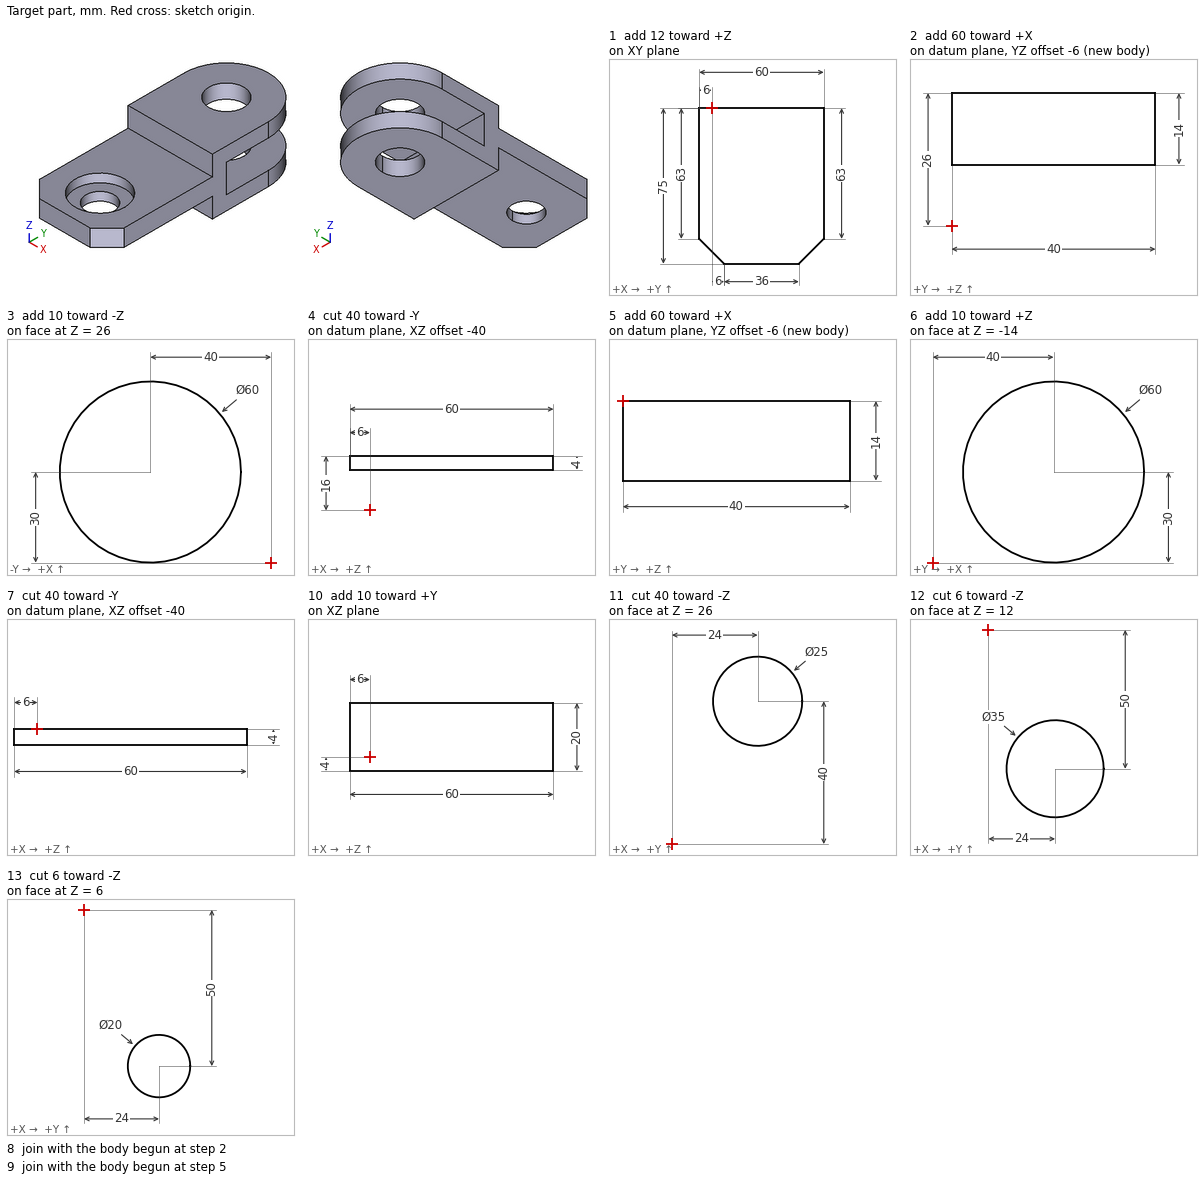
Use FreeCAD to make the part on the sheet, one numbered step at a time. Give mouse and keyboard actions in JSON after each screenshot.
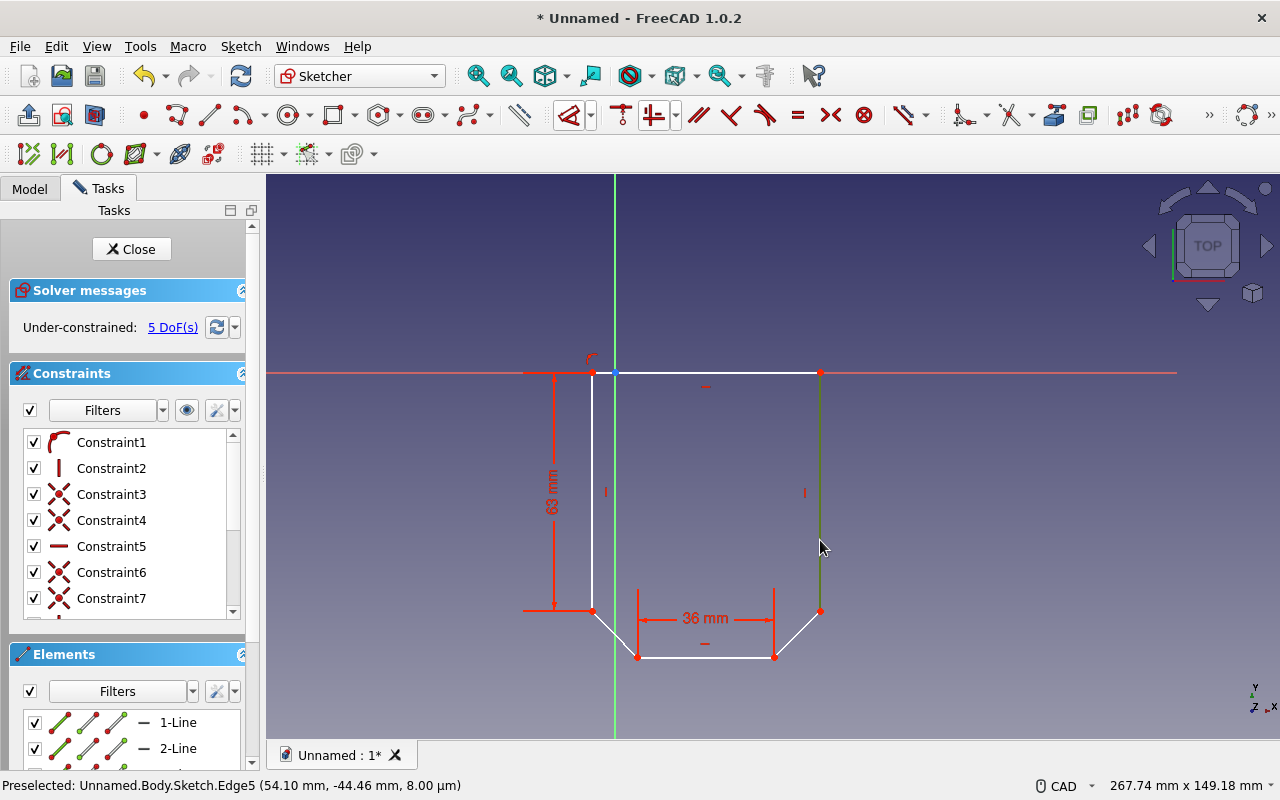
{"action": "left_click", "coordinate": [590, 116]}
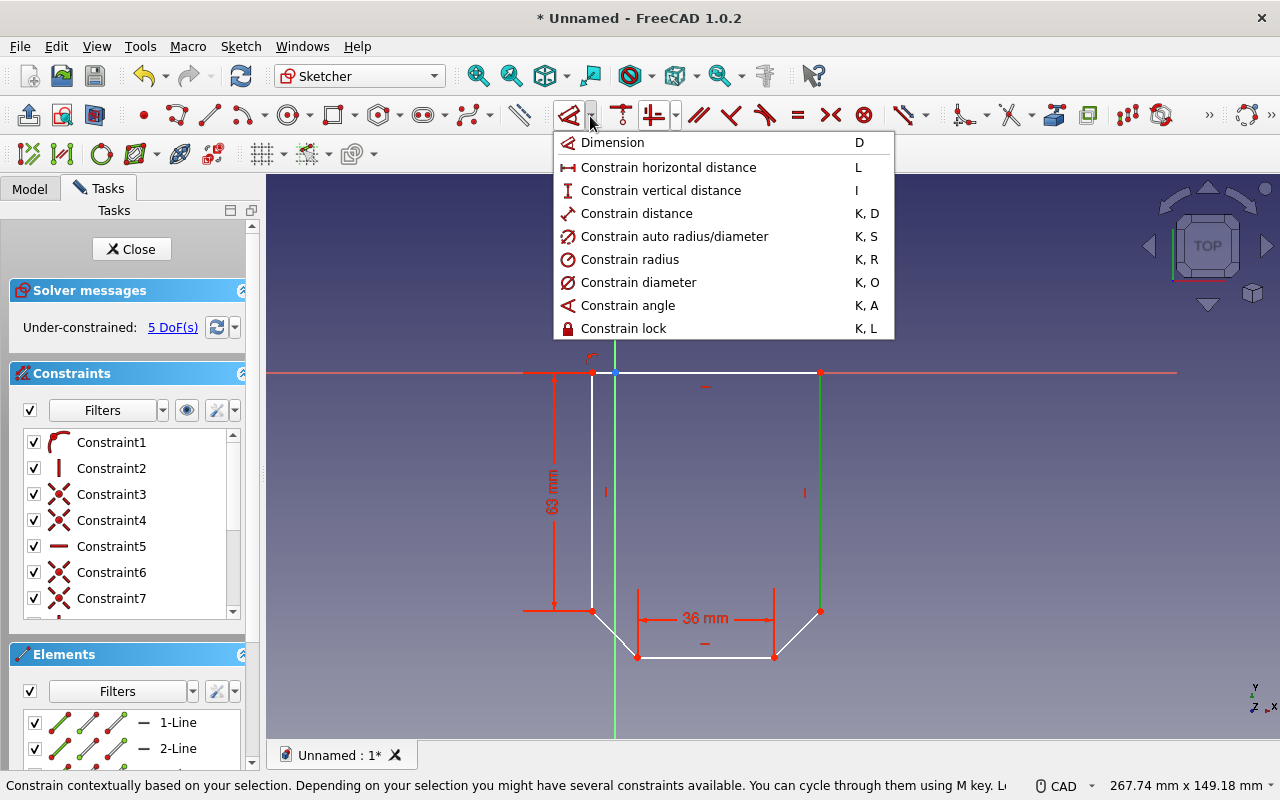
{"action": "left_click", "coordinate": [724, 190]}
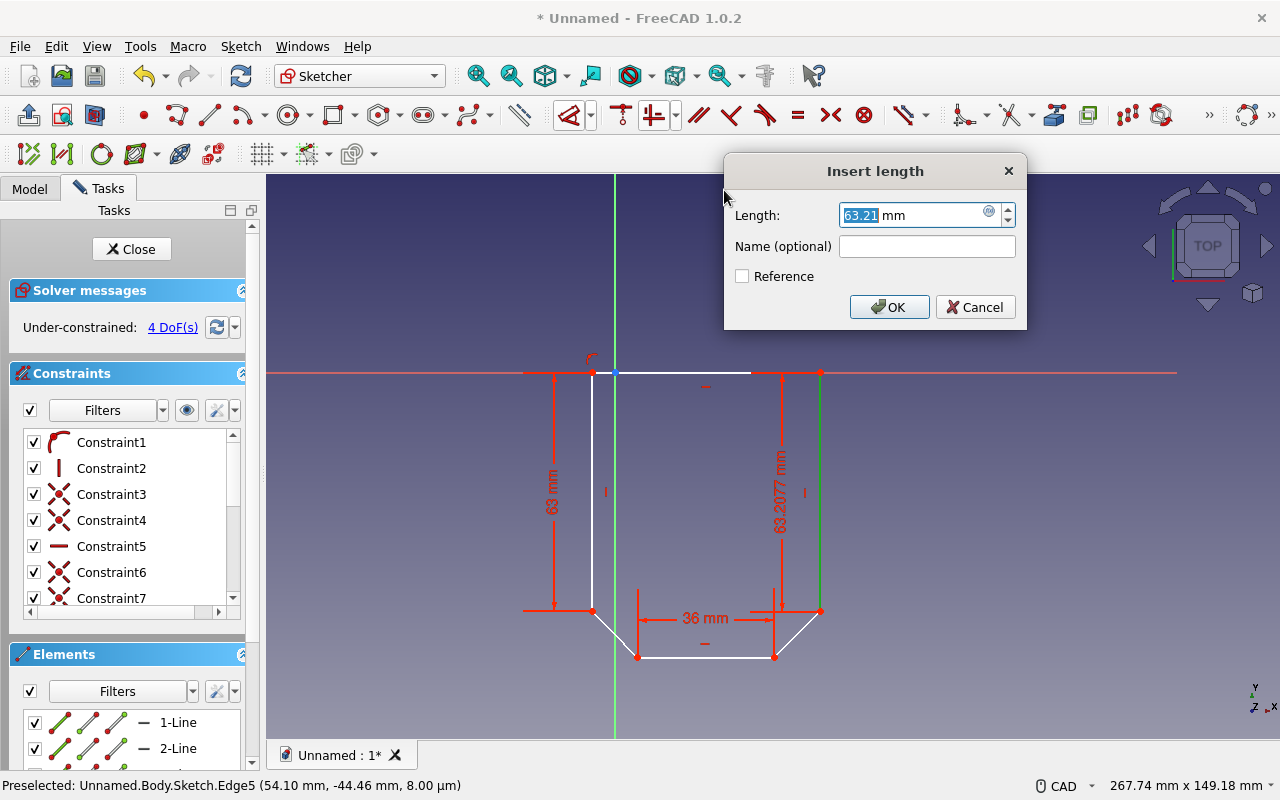
{"action": "type", "text": "63"}
{"action": "key", "text": "Return"}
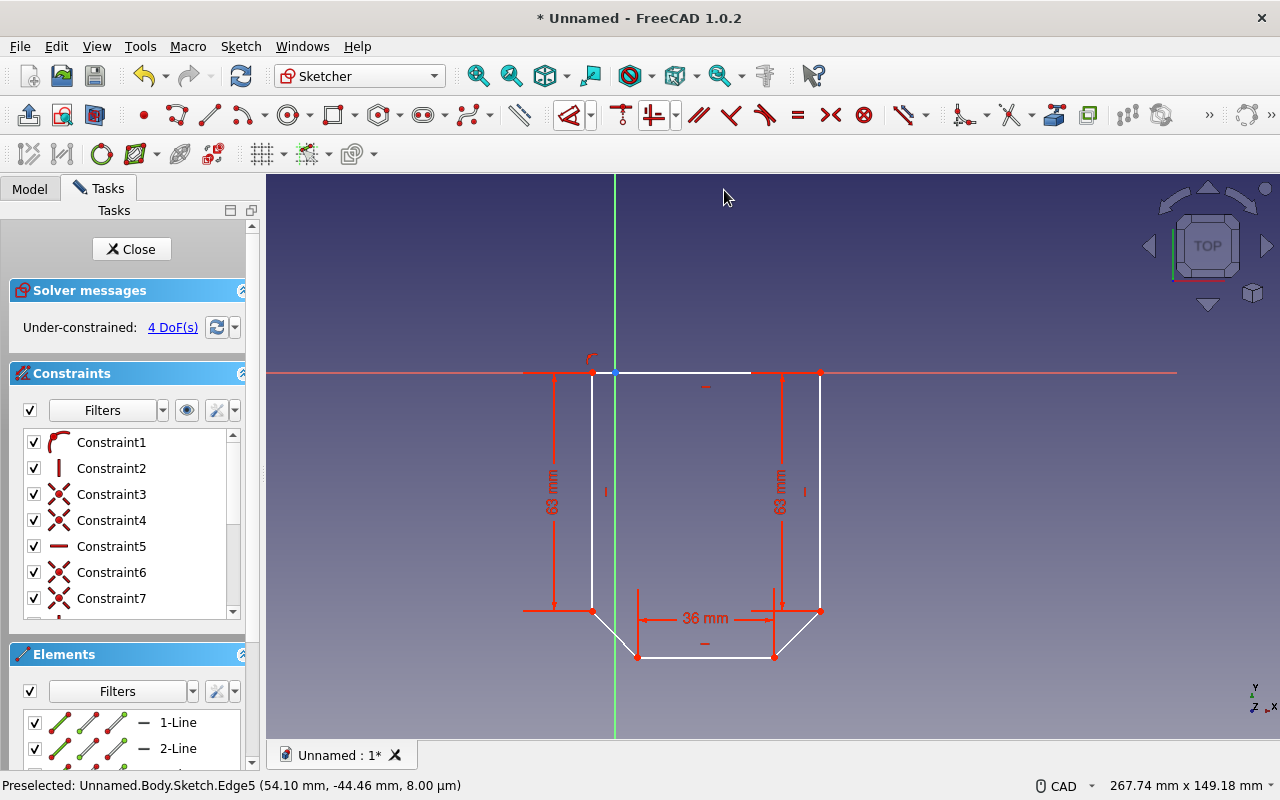
{"action": "left_click", "coordinate": [752, 373]}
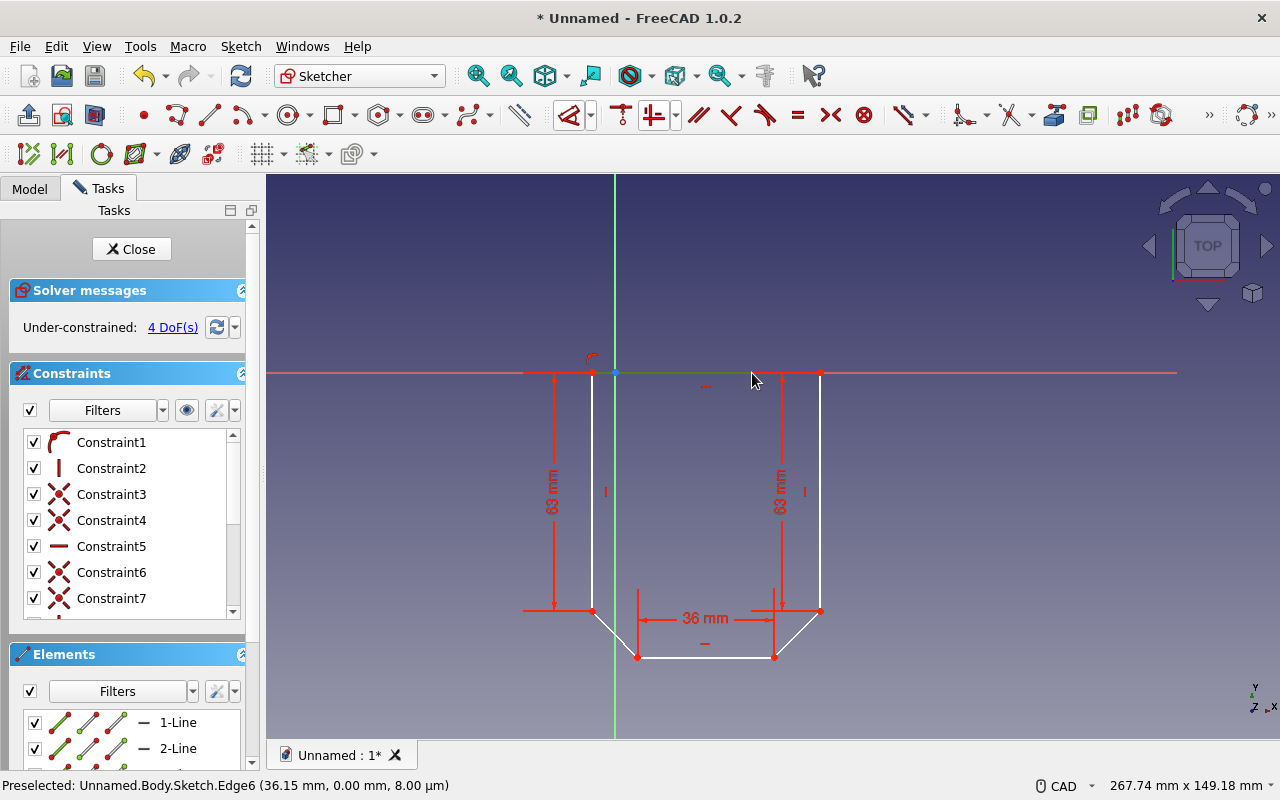
{"action": "left_click", "coordinate": [590, 116]}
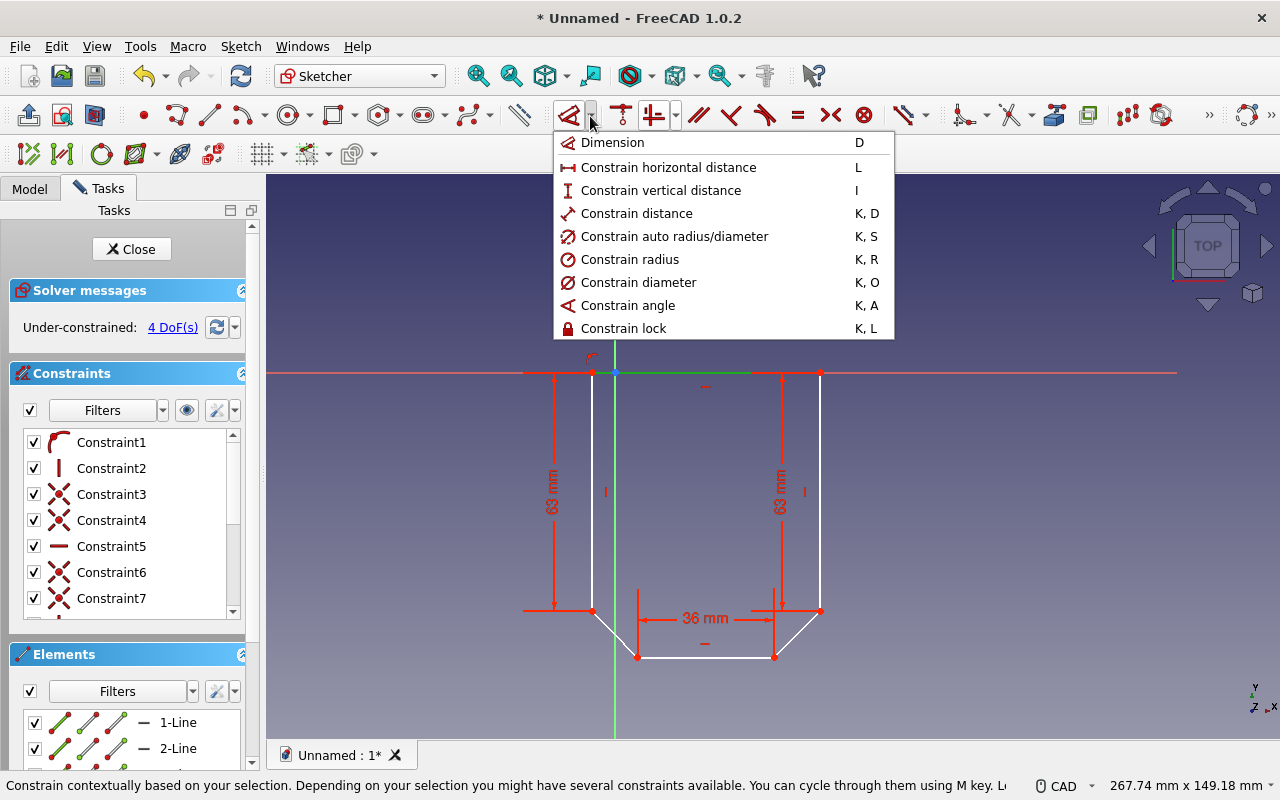
{"action": "left_click", "coordinate": [724, 168]}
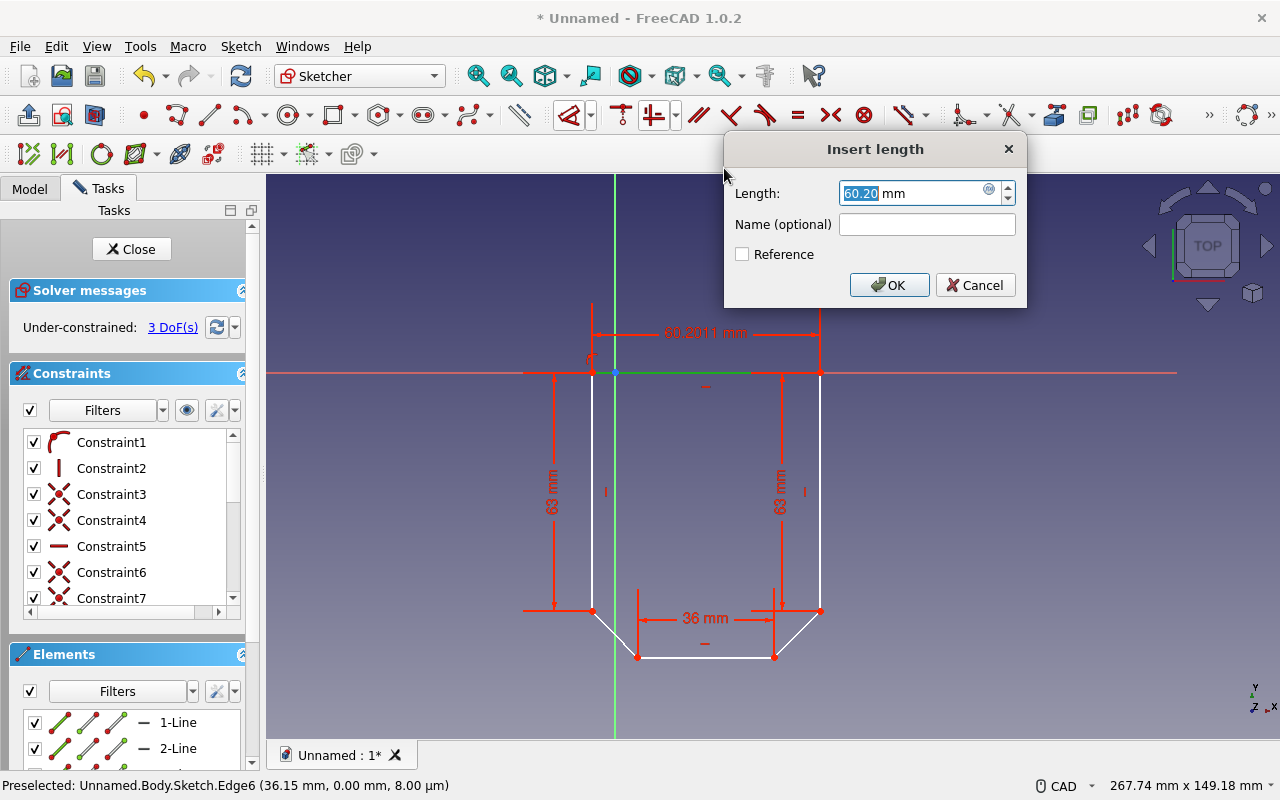
{"action": "type", "text": "60"}
{"action": "key", "text": "Return"}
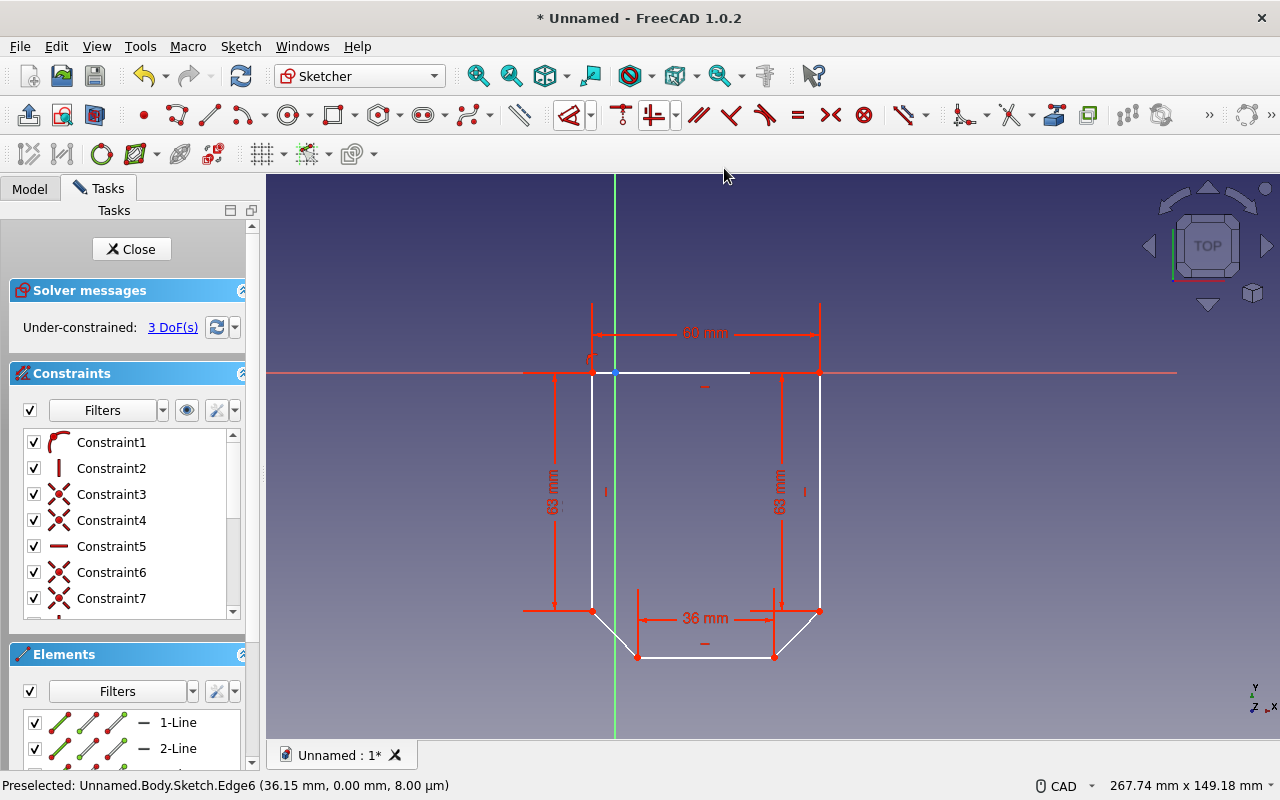
{"action": "scroll", "coordinate": [592, 373], "scroll_direction": "up", "scroll_amount": 3}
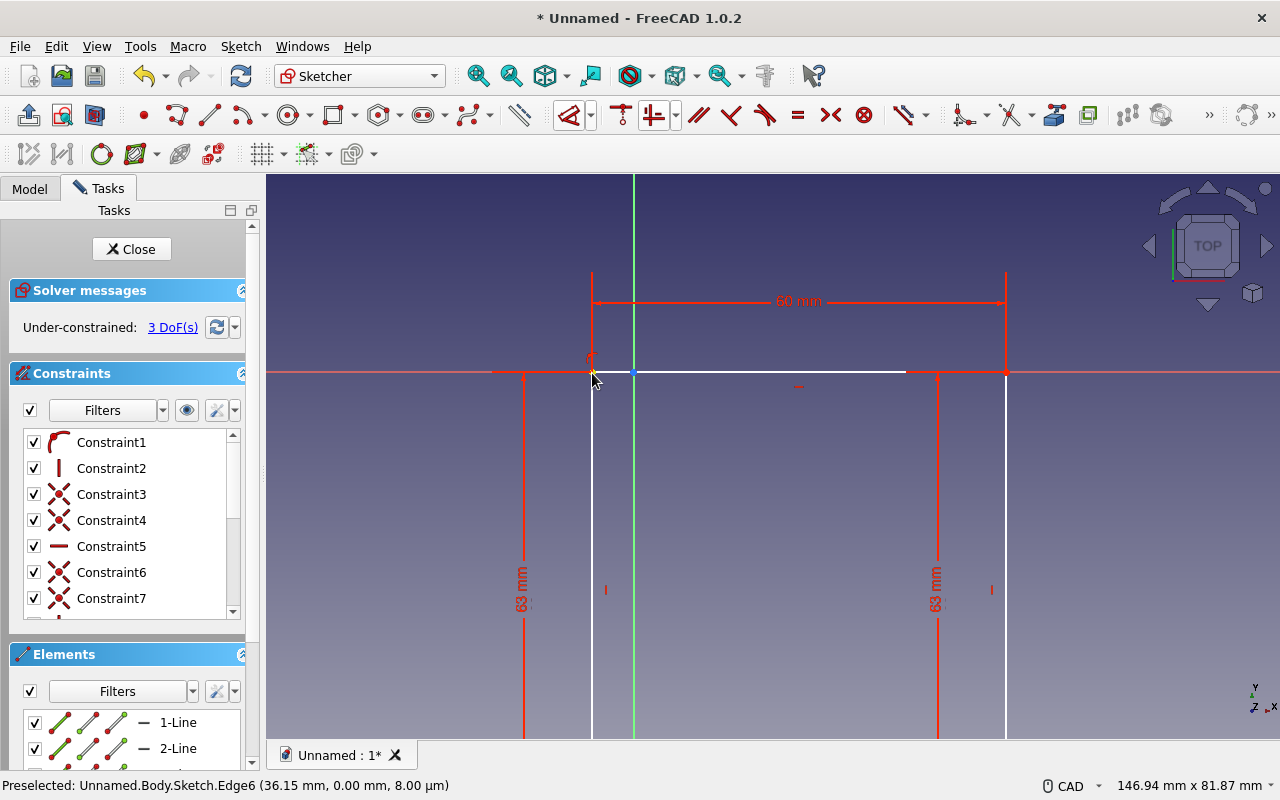
{"action": "left_click", "coordinate": [592, 372]}